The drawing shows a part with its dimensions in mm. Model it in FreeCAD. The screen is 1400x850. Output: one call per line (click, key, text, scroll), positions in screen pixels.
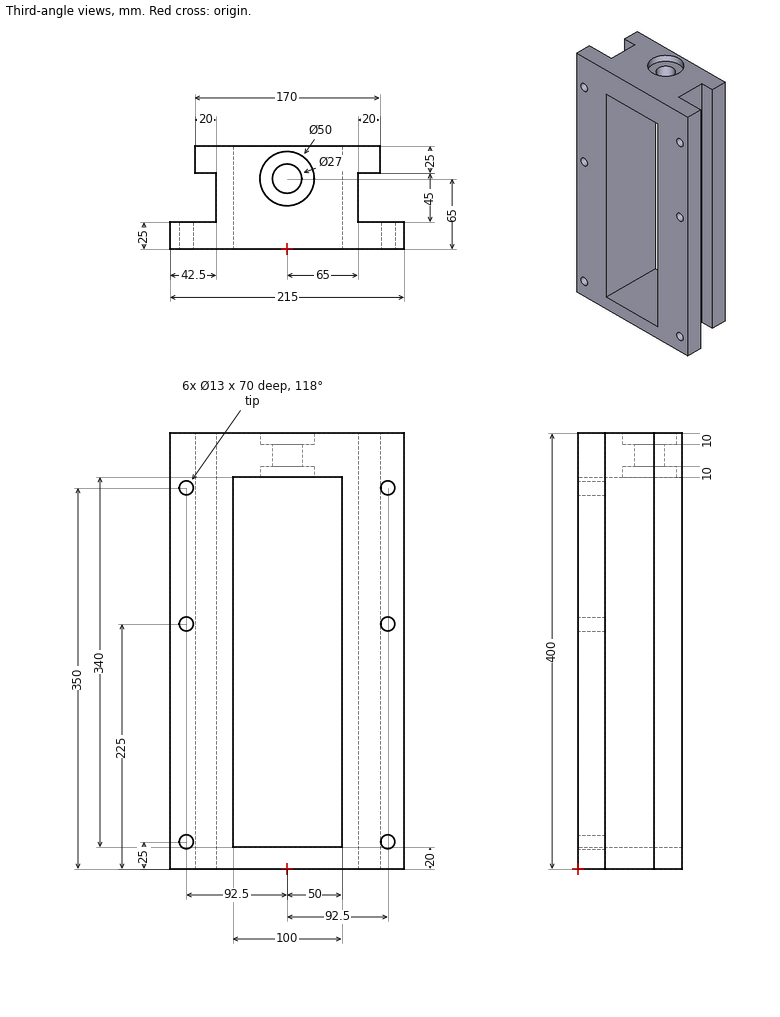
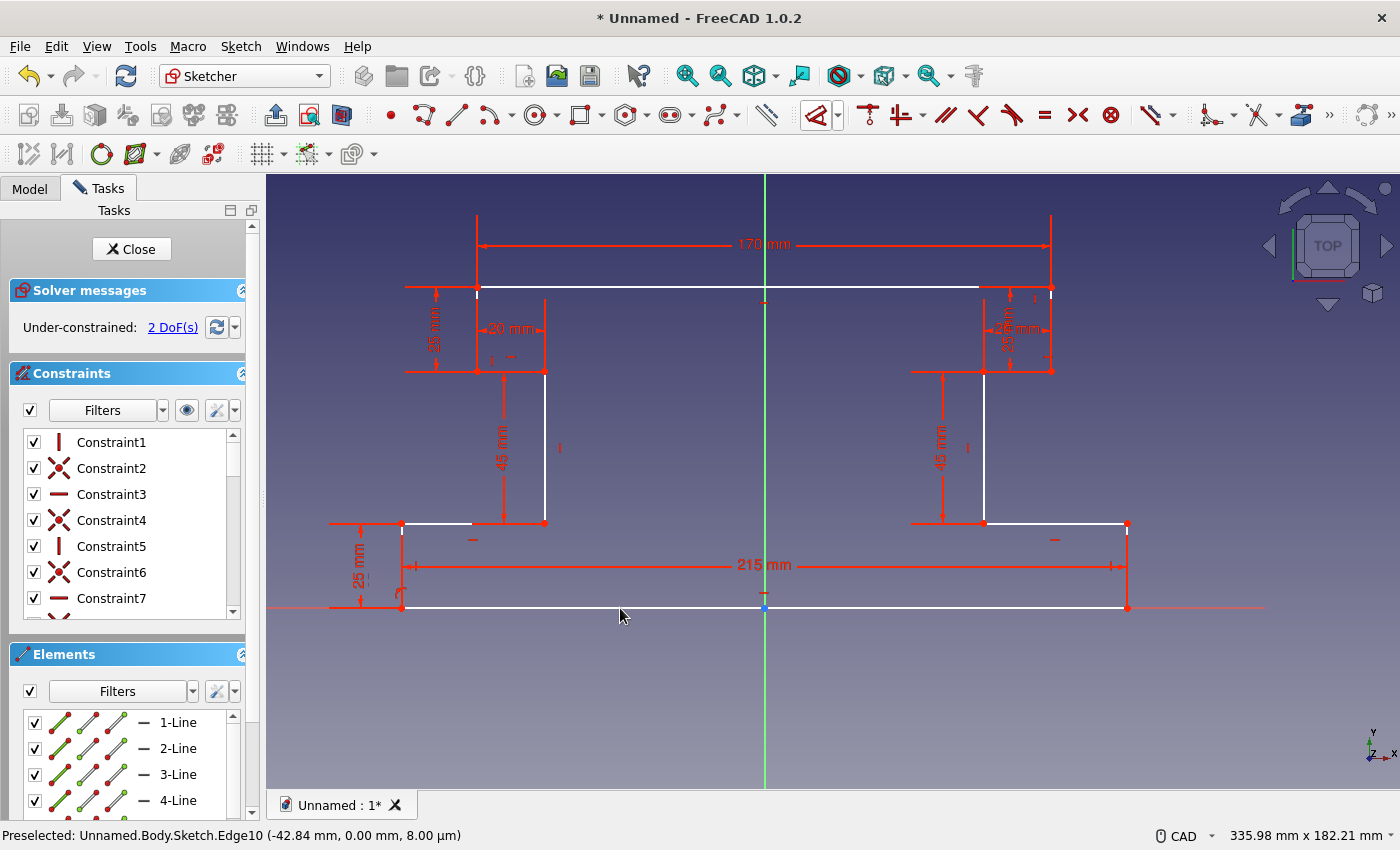
click(984, 524)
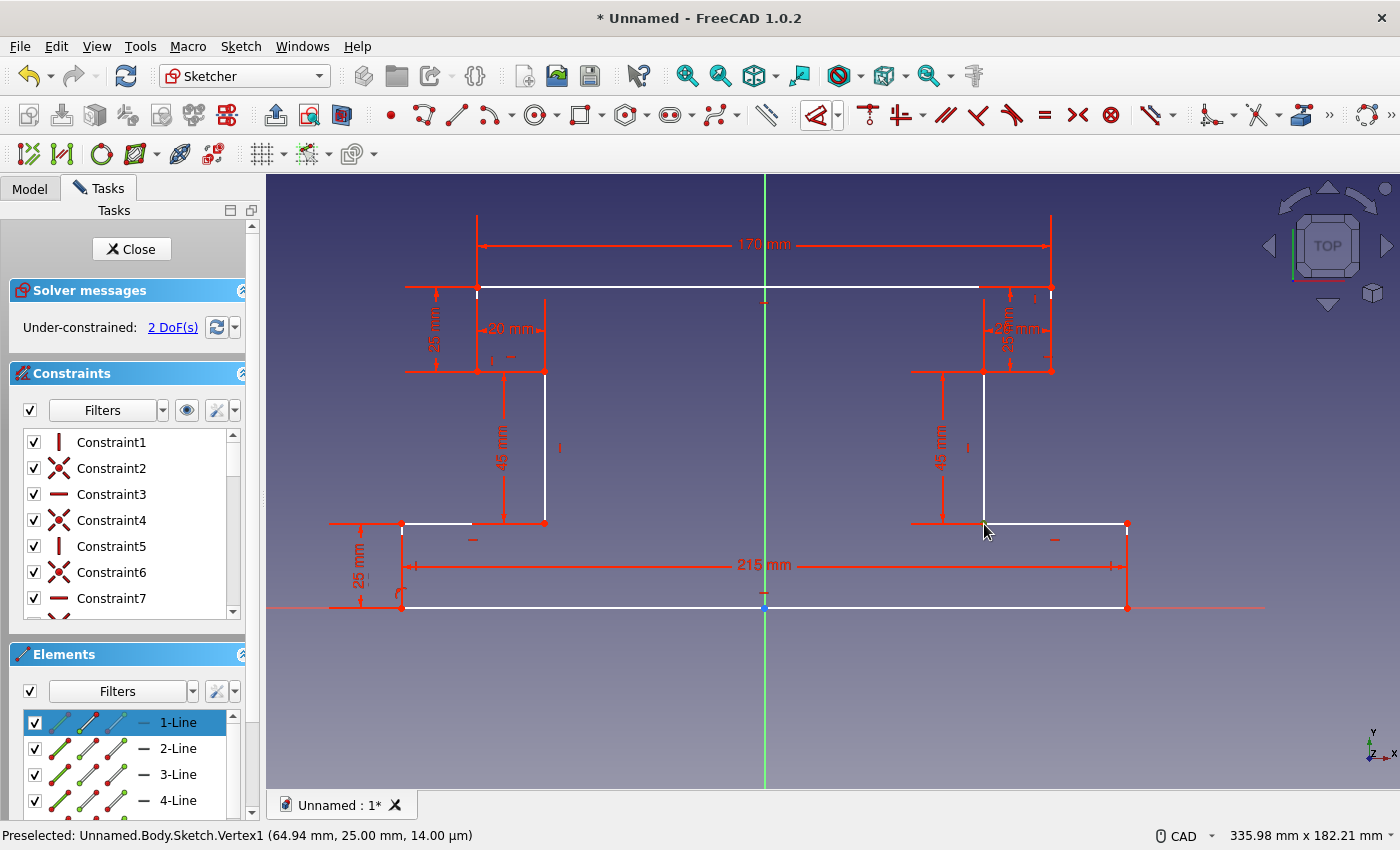
key(l)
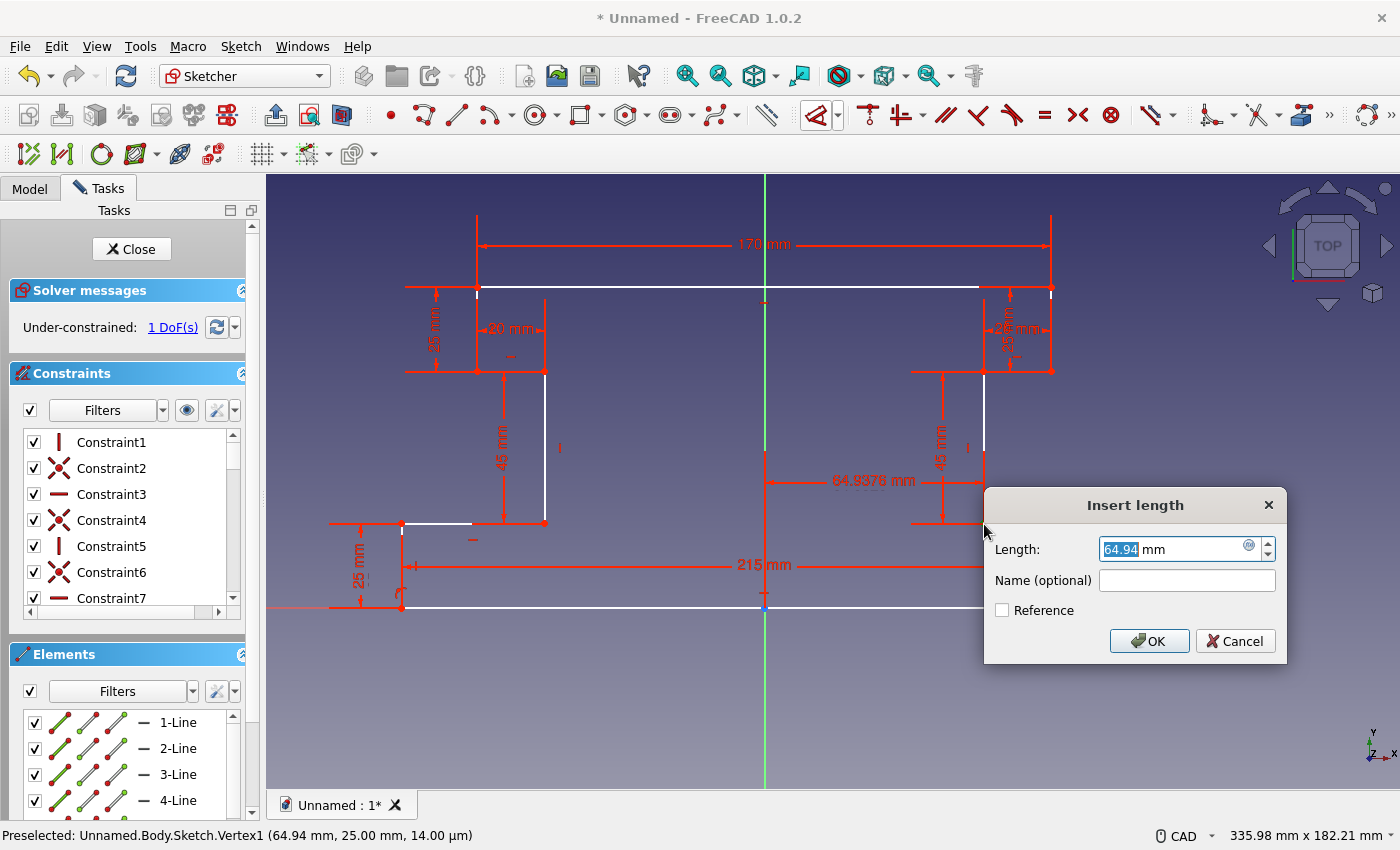
text(65)
key(Return)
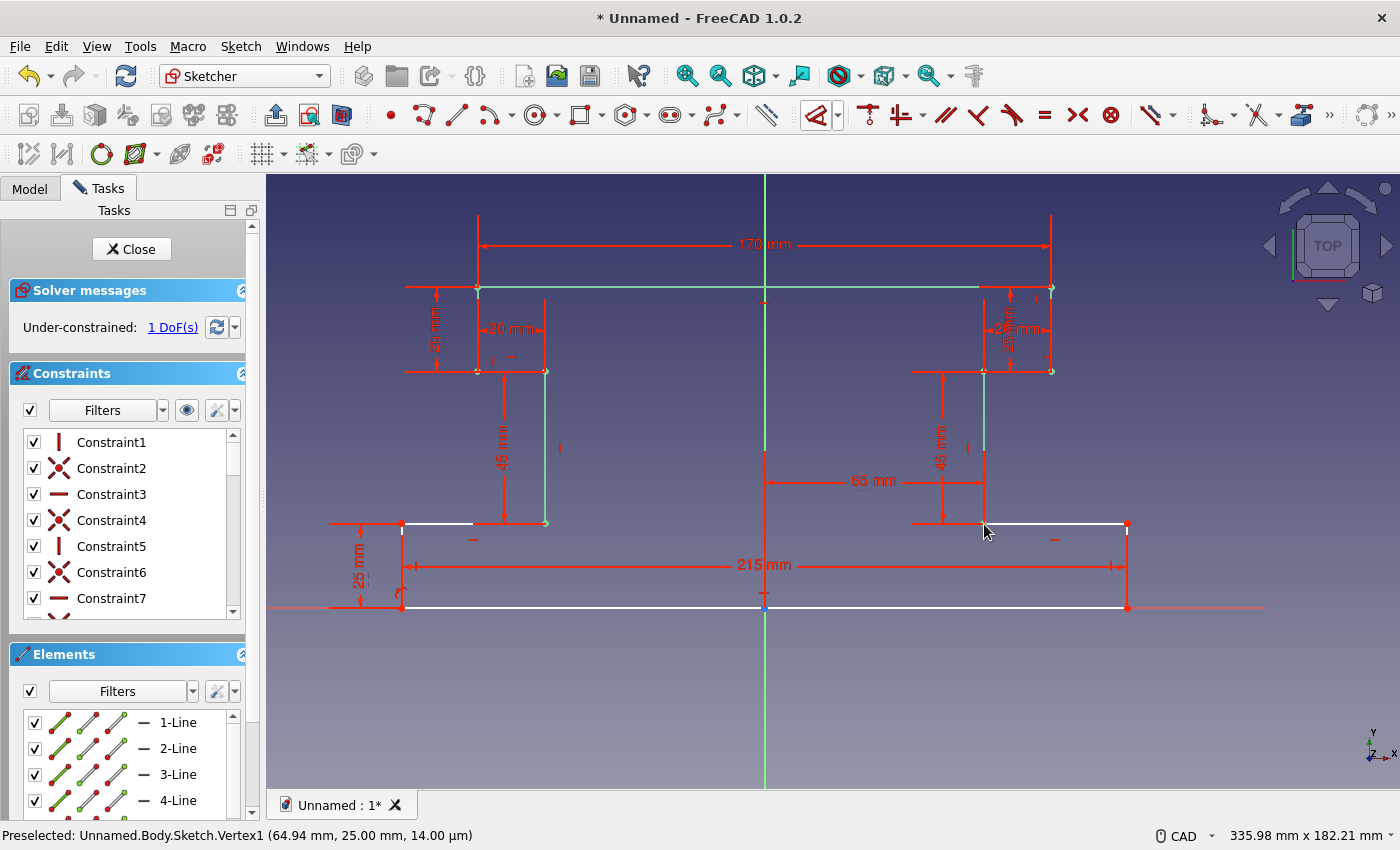
click(502, 524)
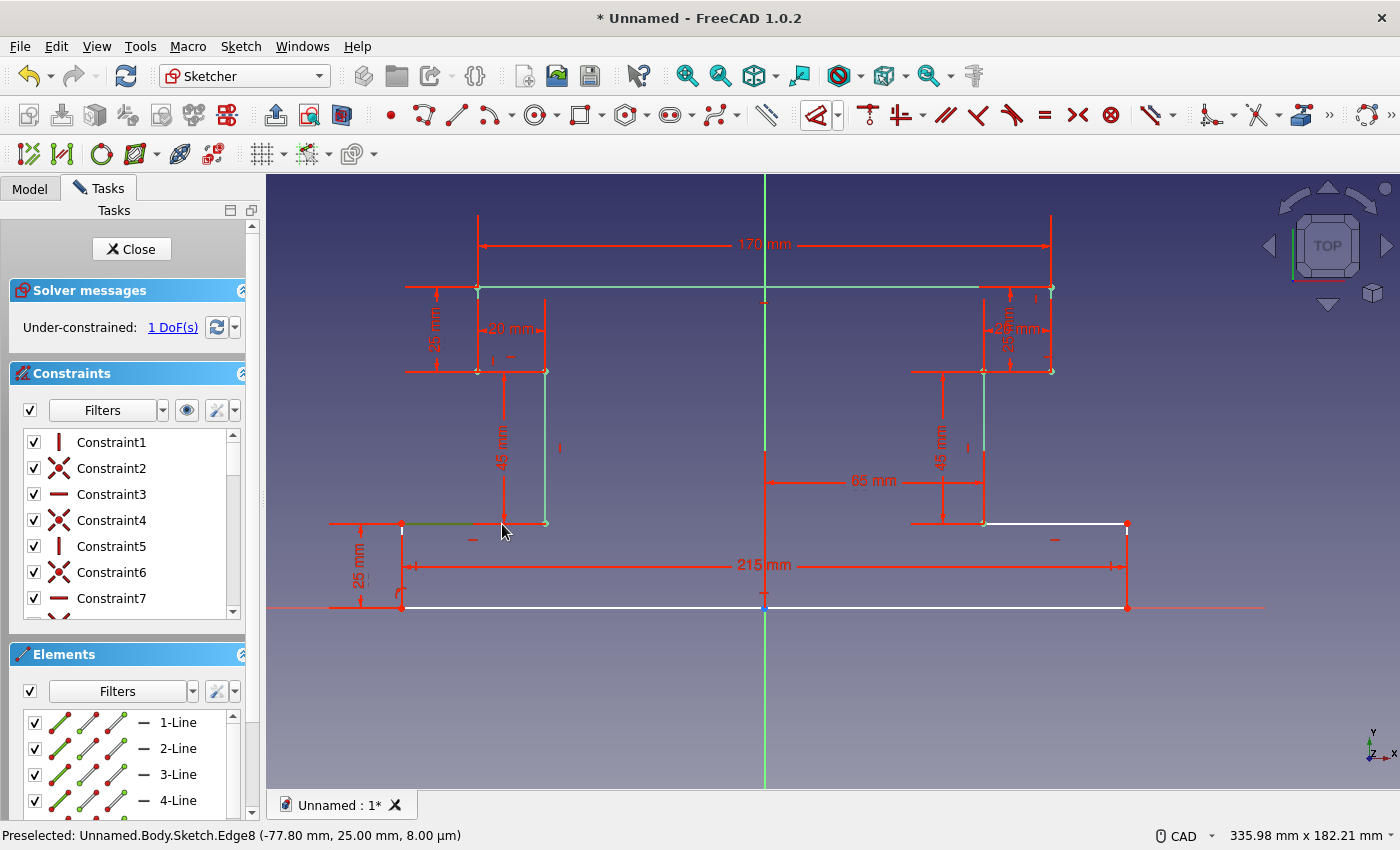
key(l)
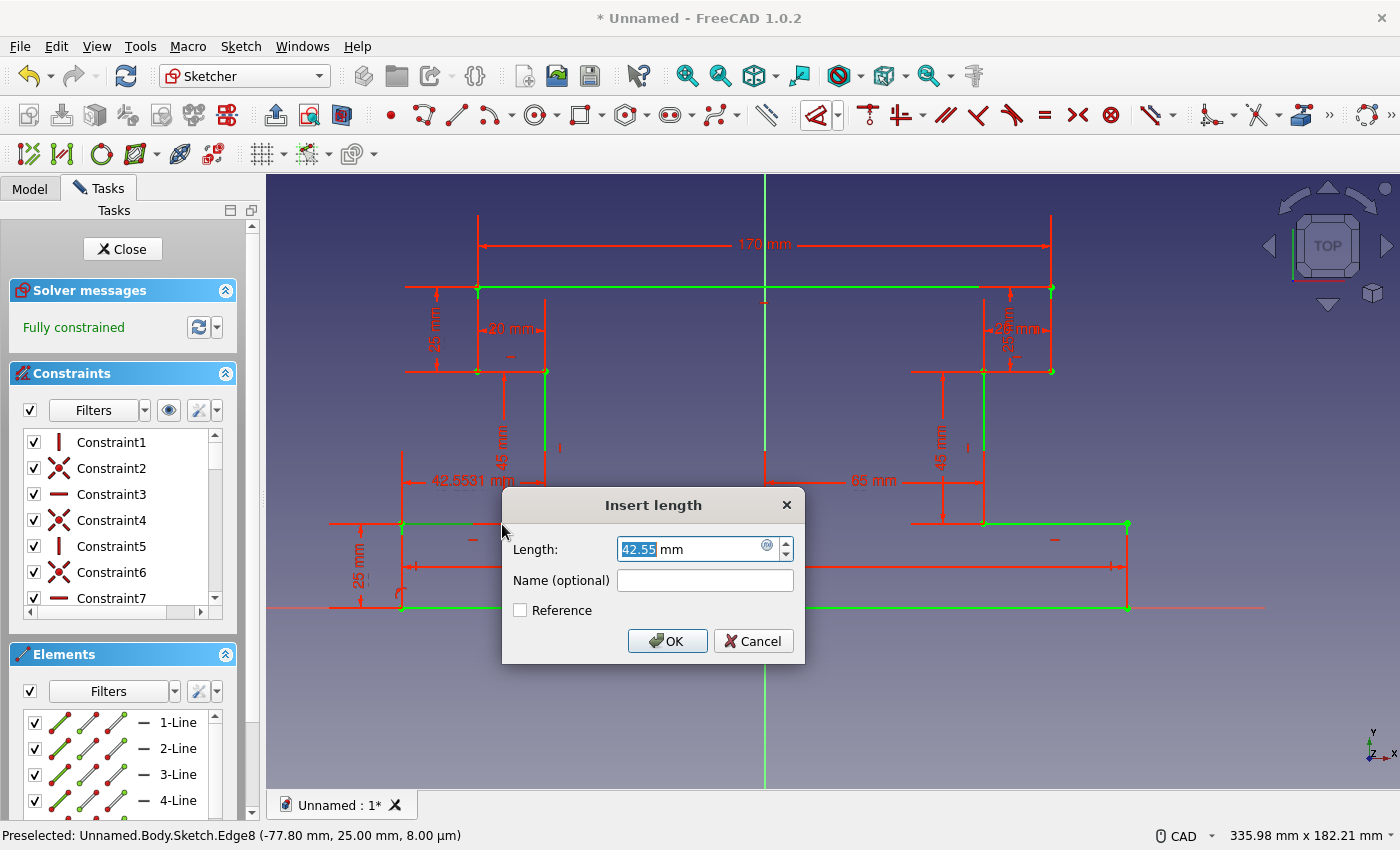
text(42.5)
key(Return)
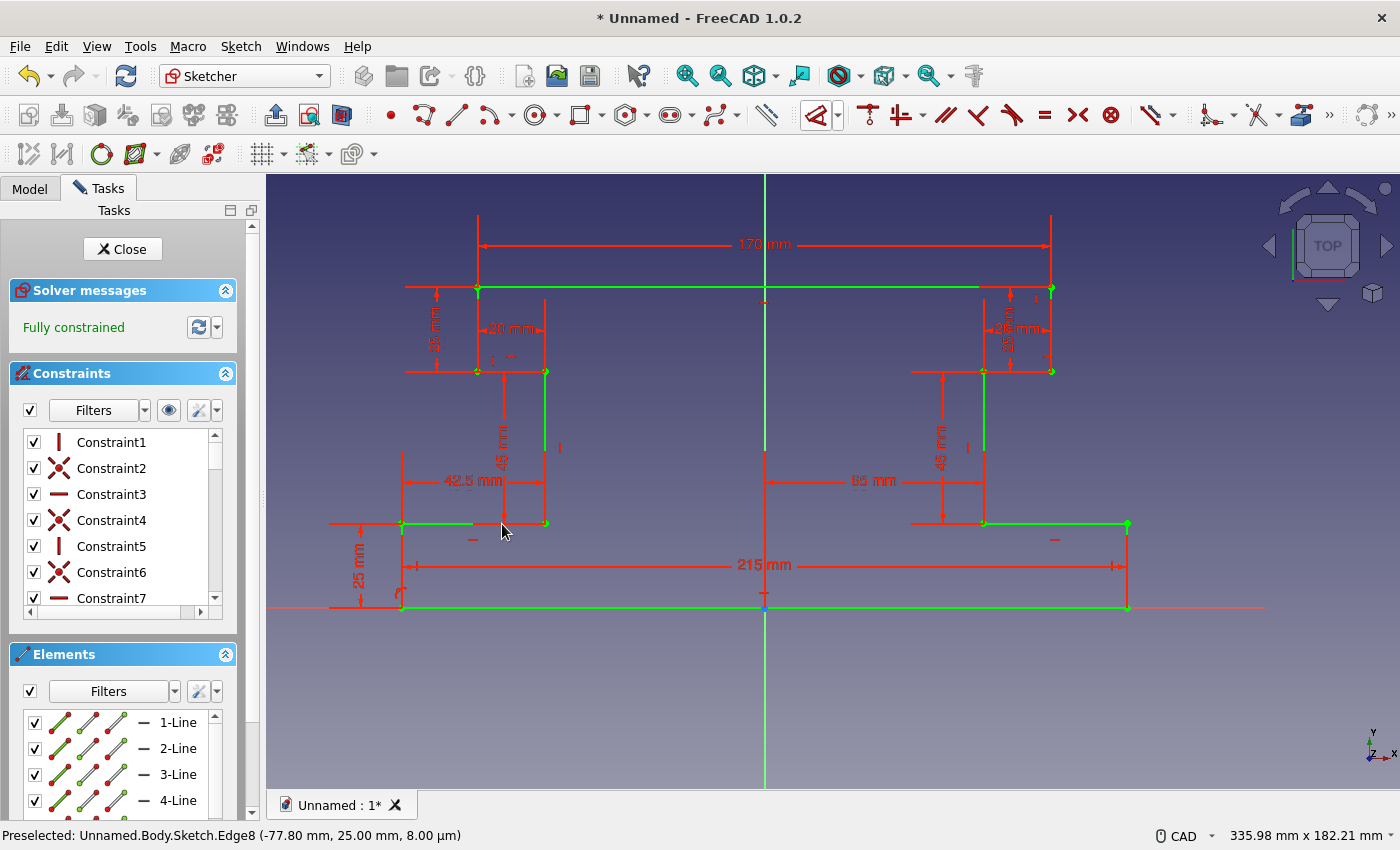
click(123, 249)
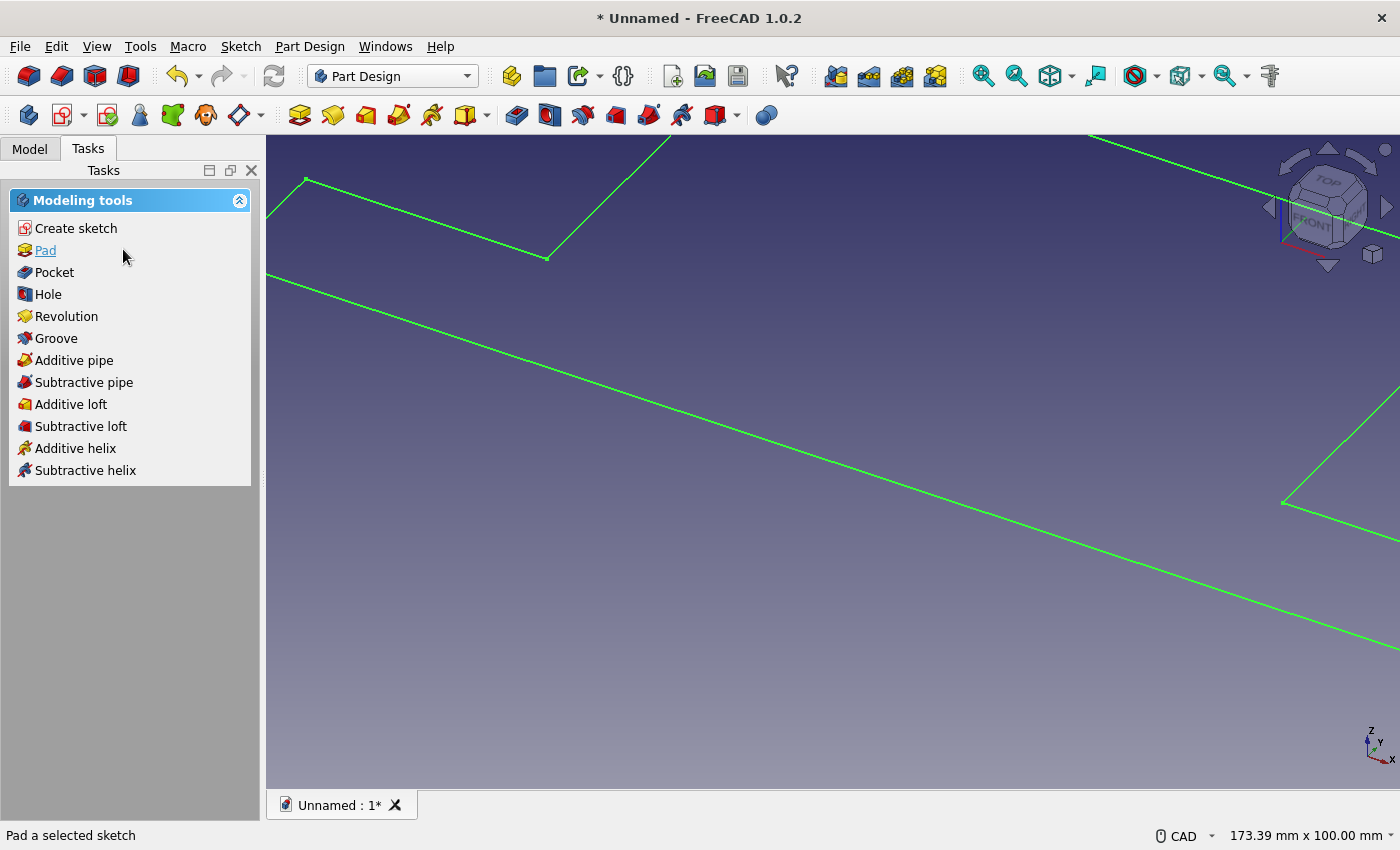
click(300, 116)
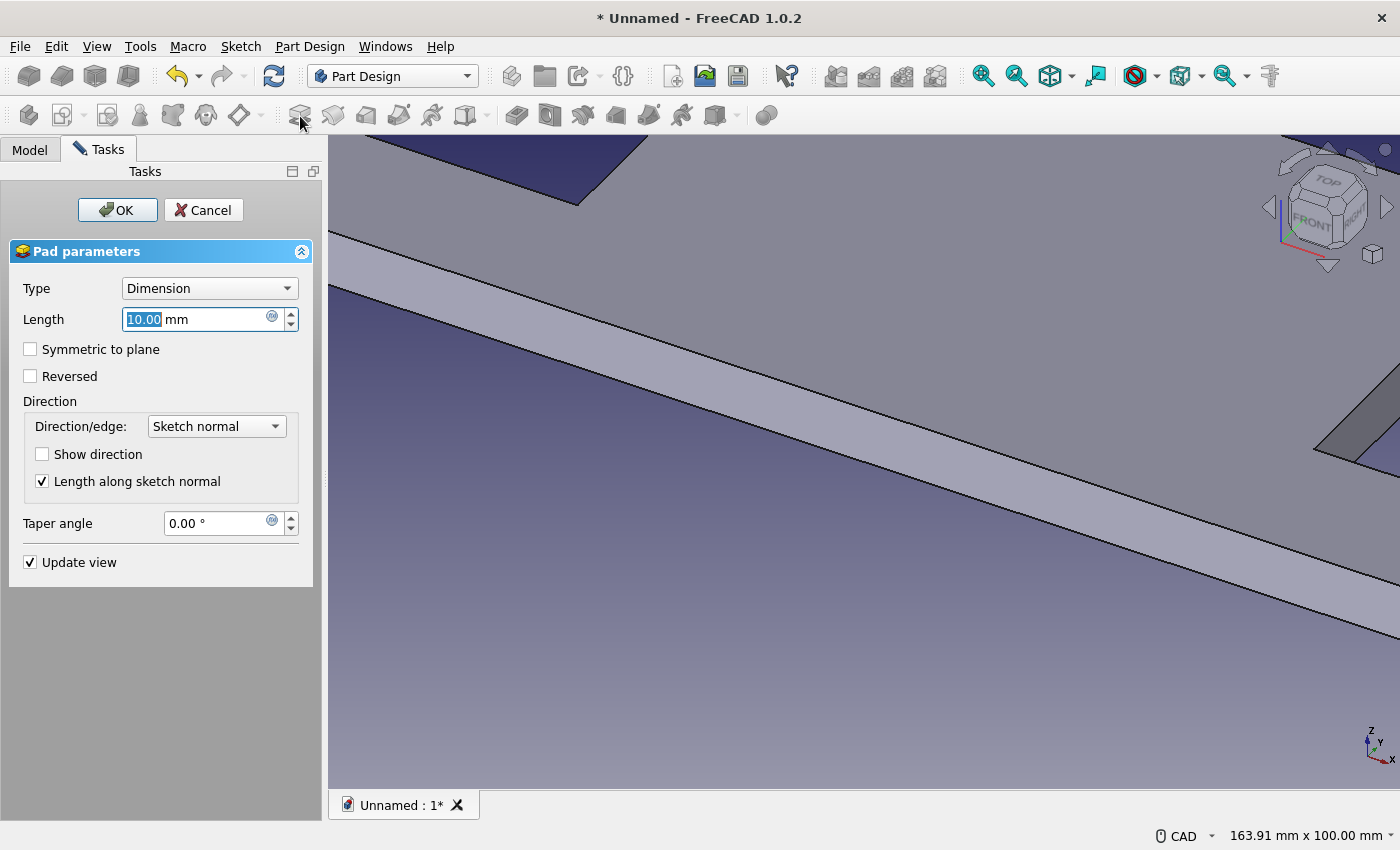
text(400)
key(Tab)